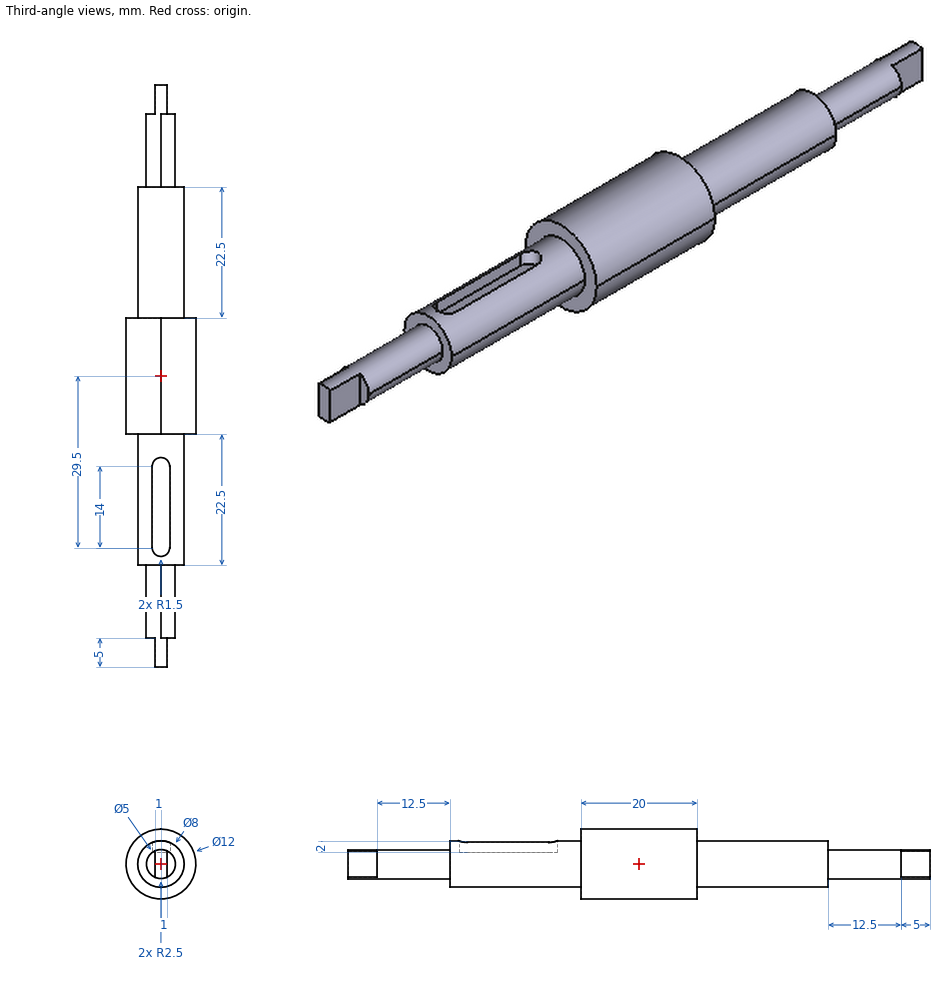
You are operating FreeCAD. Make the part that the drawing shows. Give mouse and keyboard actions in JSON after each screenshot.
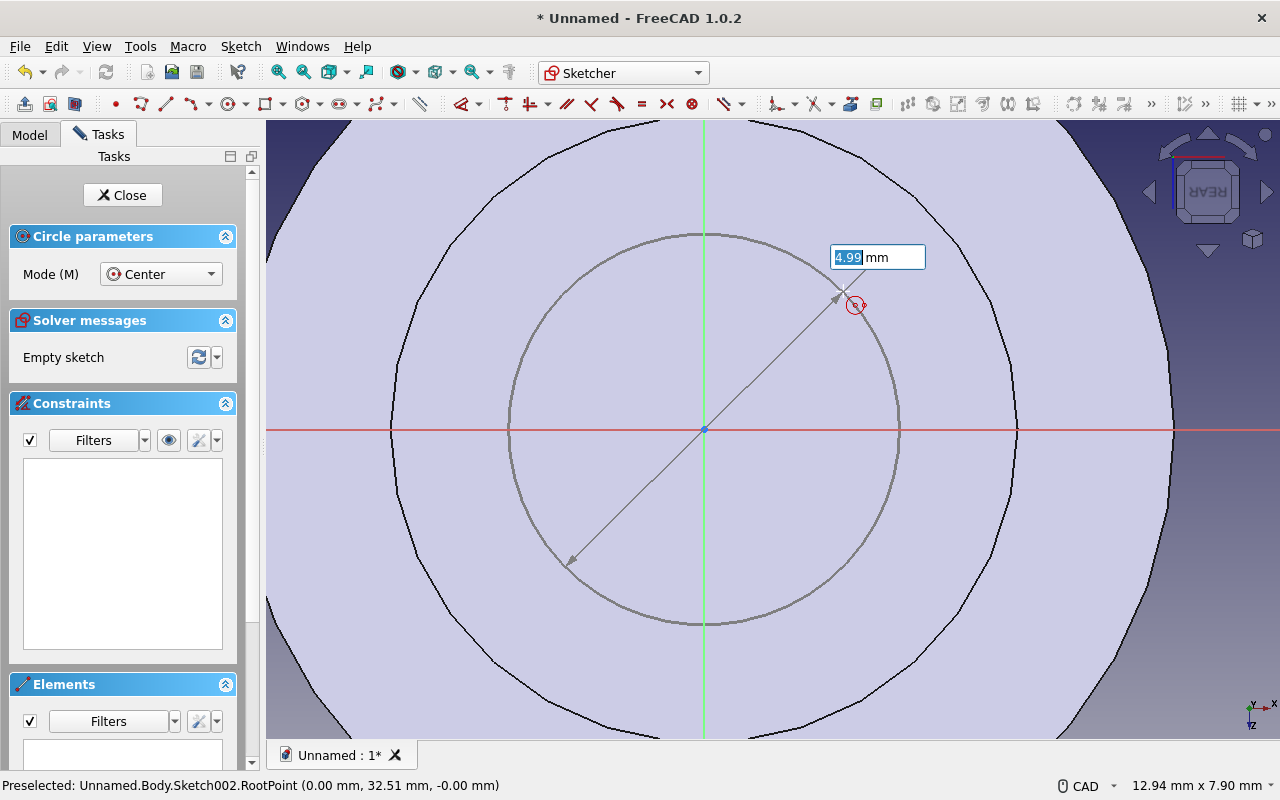
{"action": "type", "text": "5"}
{"action": "key", "text": "Return"}
{"action": "key", "text": "Escape"}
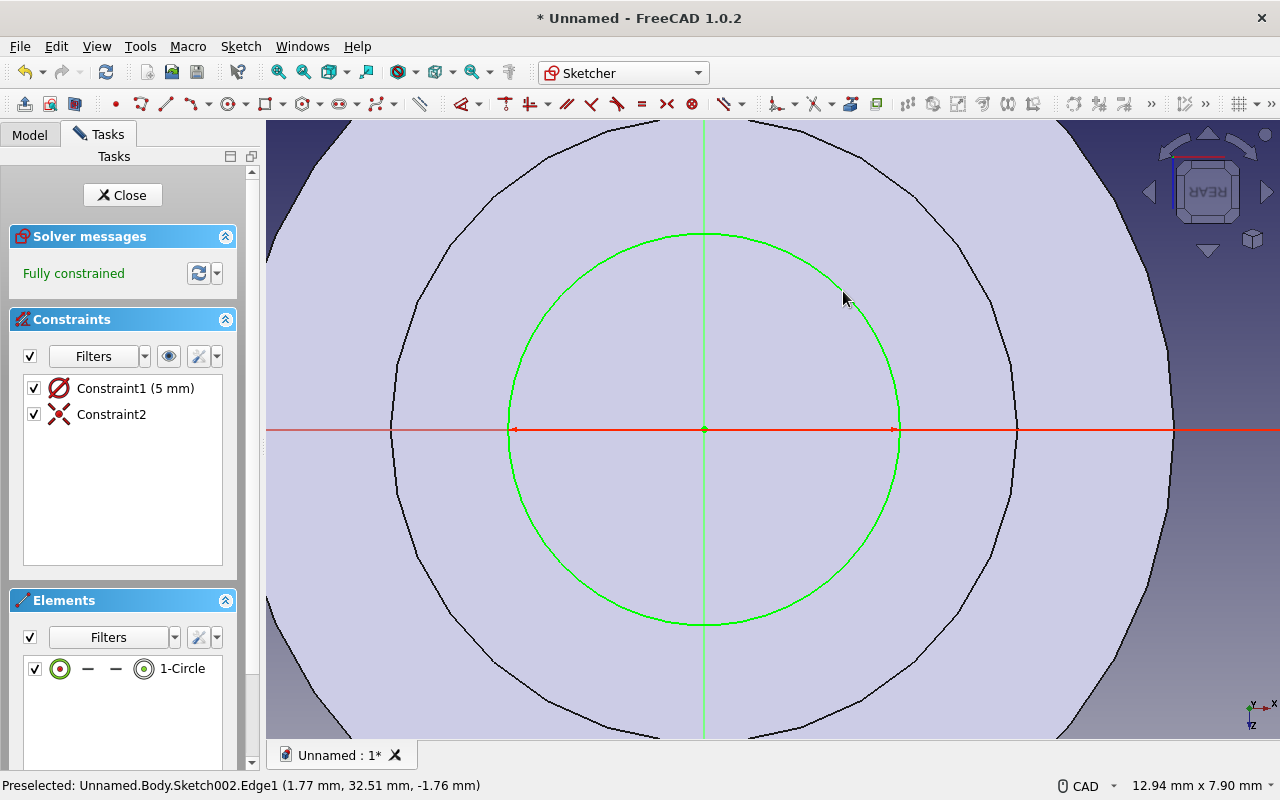
{"action": "left_click", "coordinate": [123, 195]}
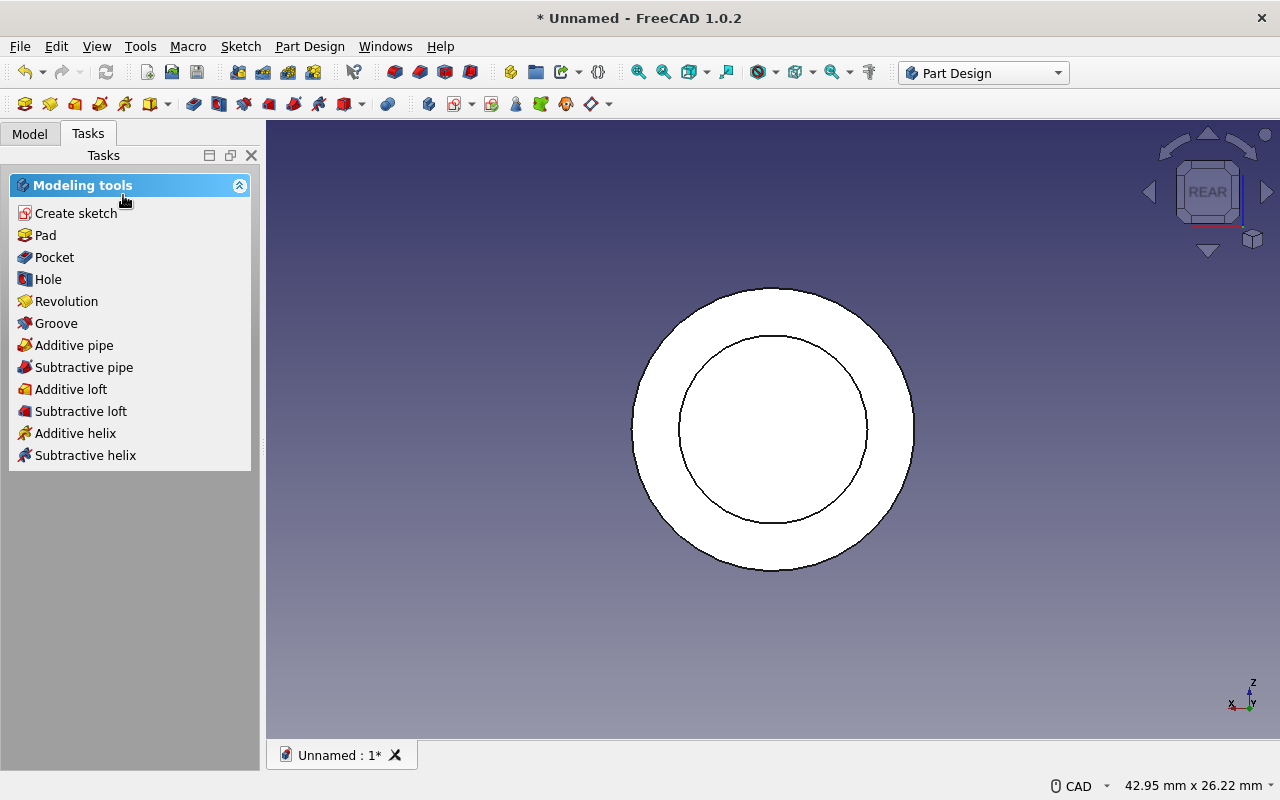
{"action": "left_click", "coordinate": [25, 104]}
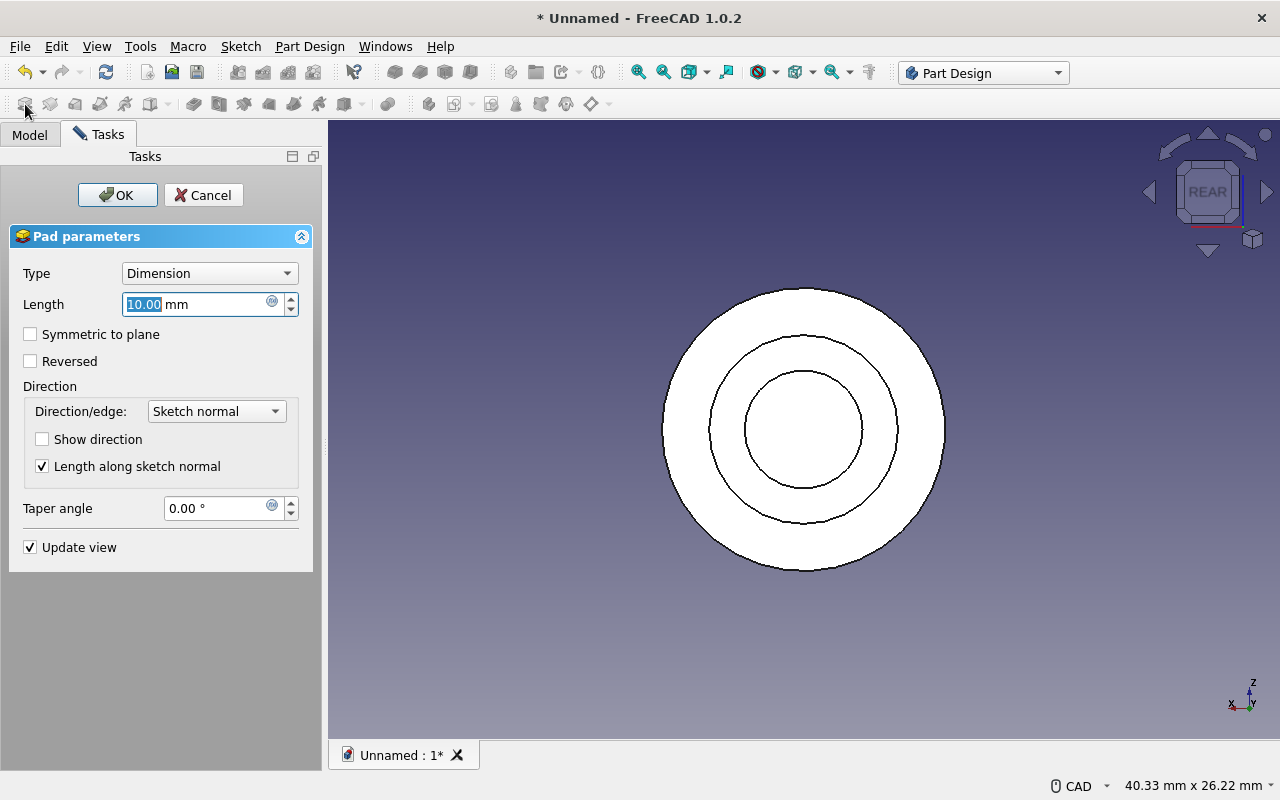
{"action": "type", "text": "12.5"}
{"action": "key", "text": "Tab"}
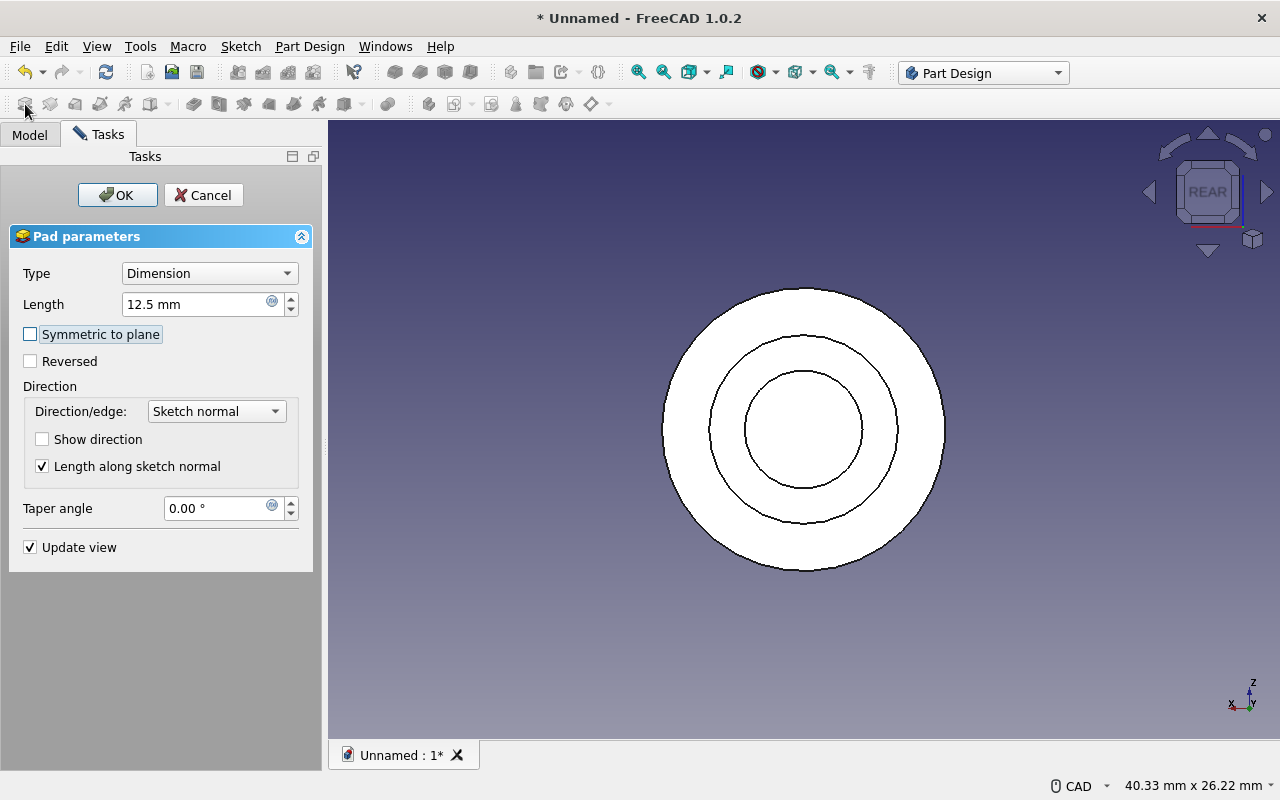
{"action": "left_click", "coordinate": [118, 195]}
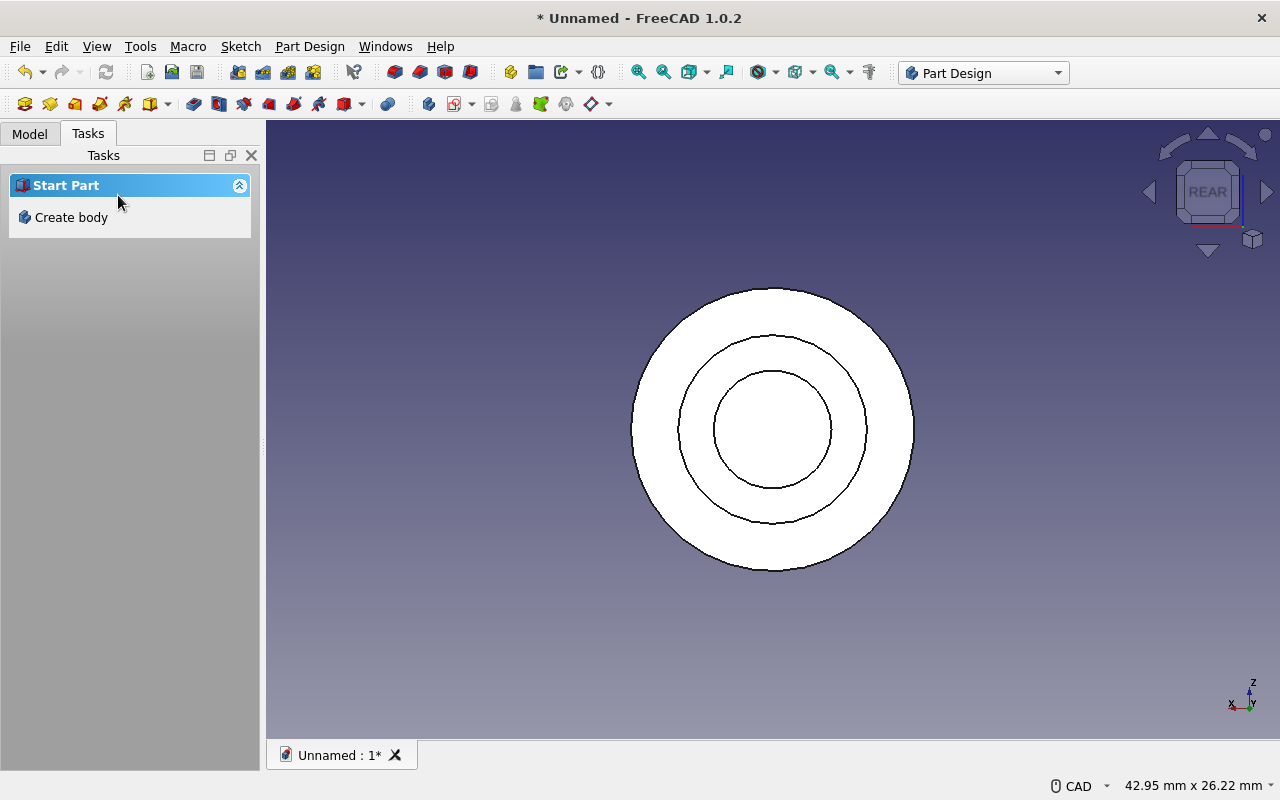
{"action": "left_click", "coordinate": [30, 134]}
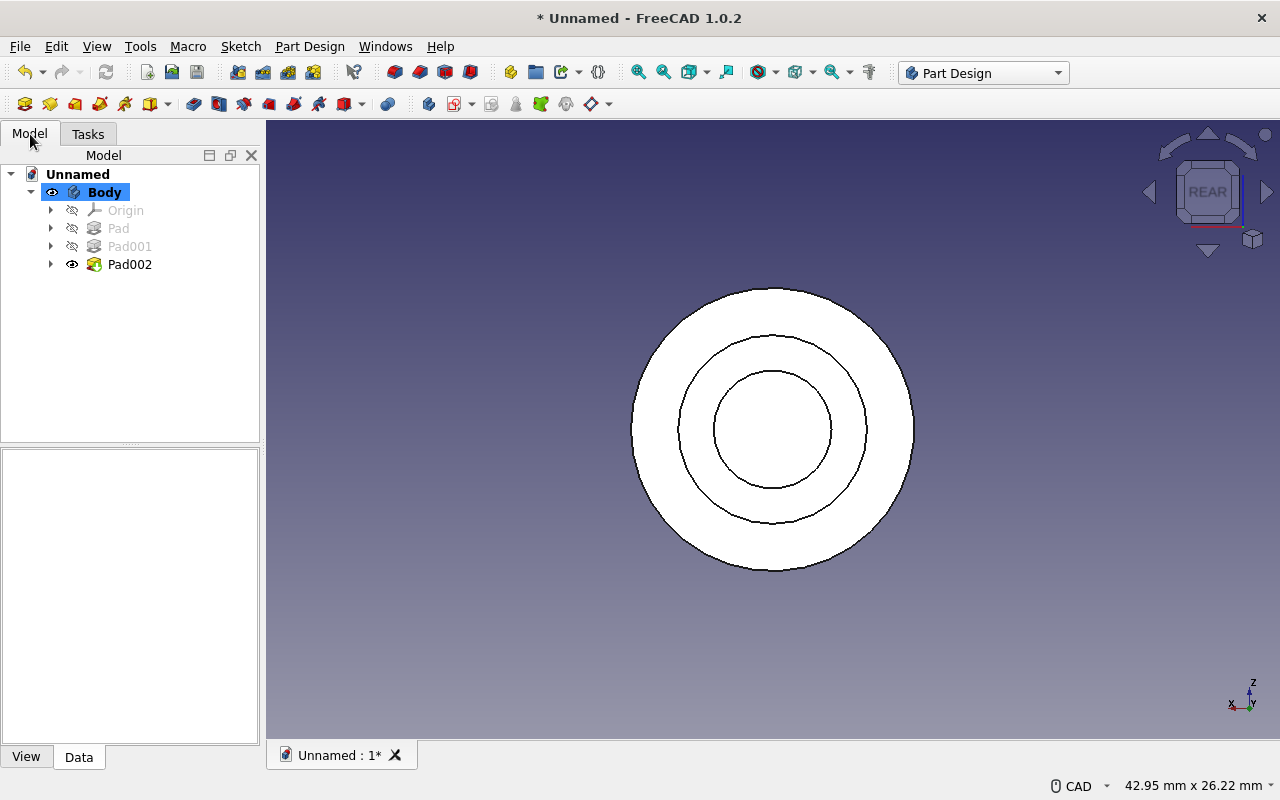
{"action": "left_click", "coordinate": [51, 210]}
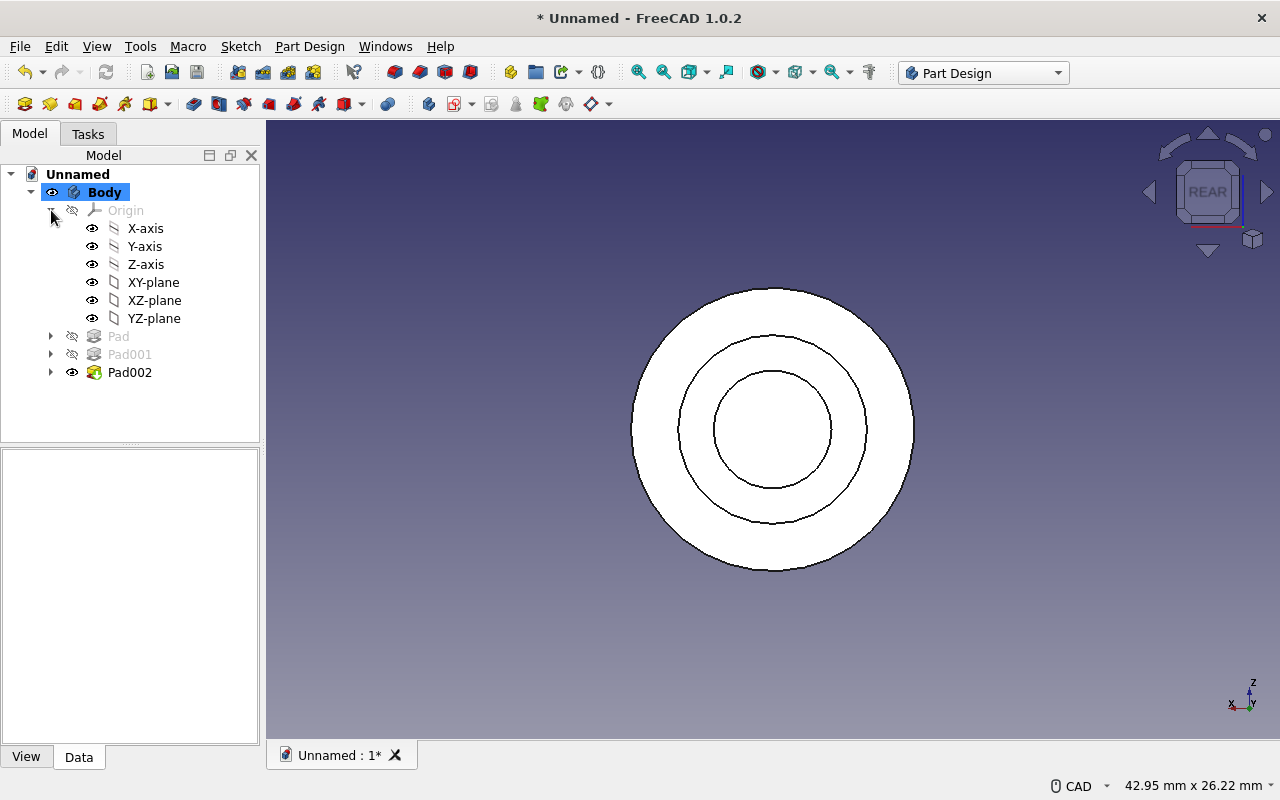
{"action": "left_click", "coordinate": [137, 300]}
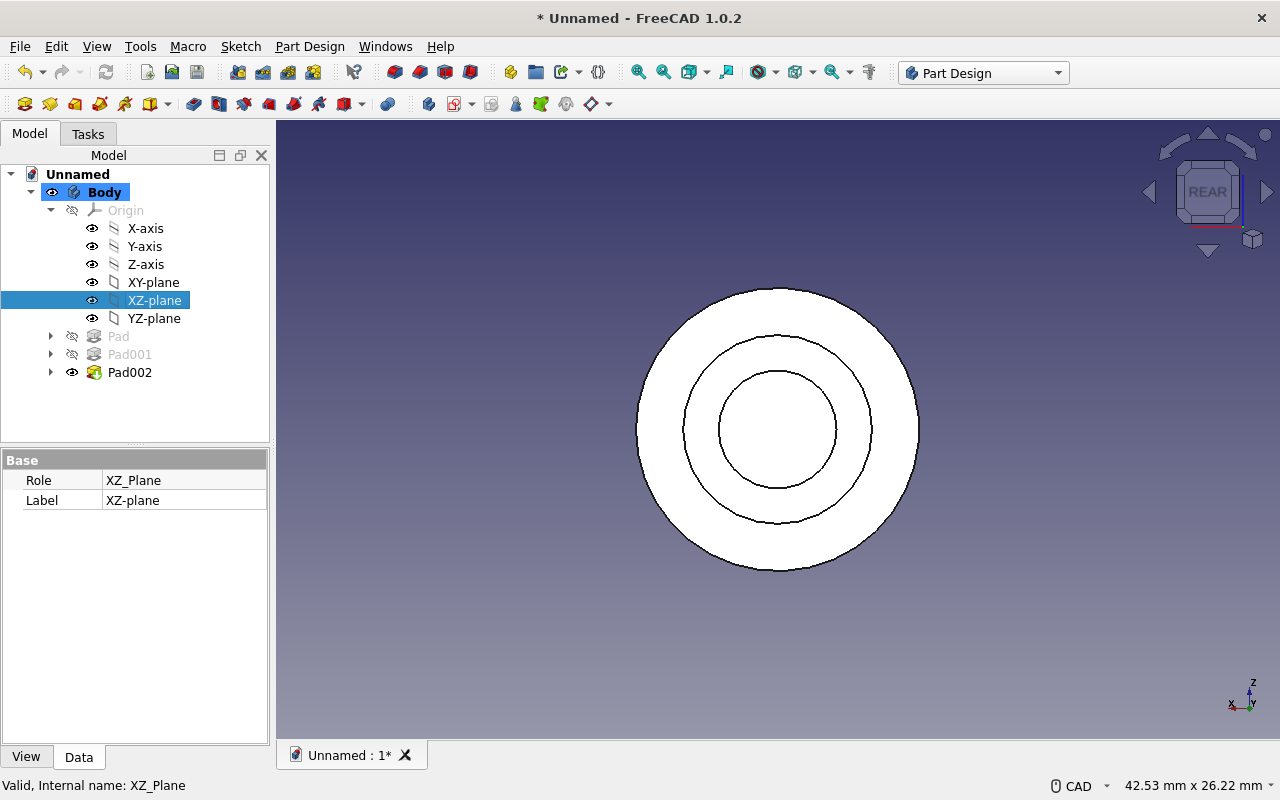
{"action": "left_click", "coordinate": [590, 104]}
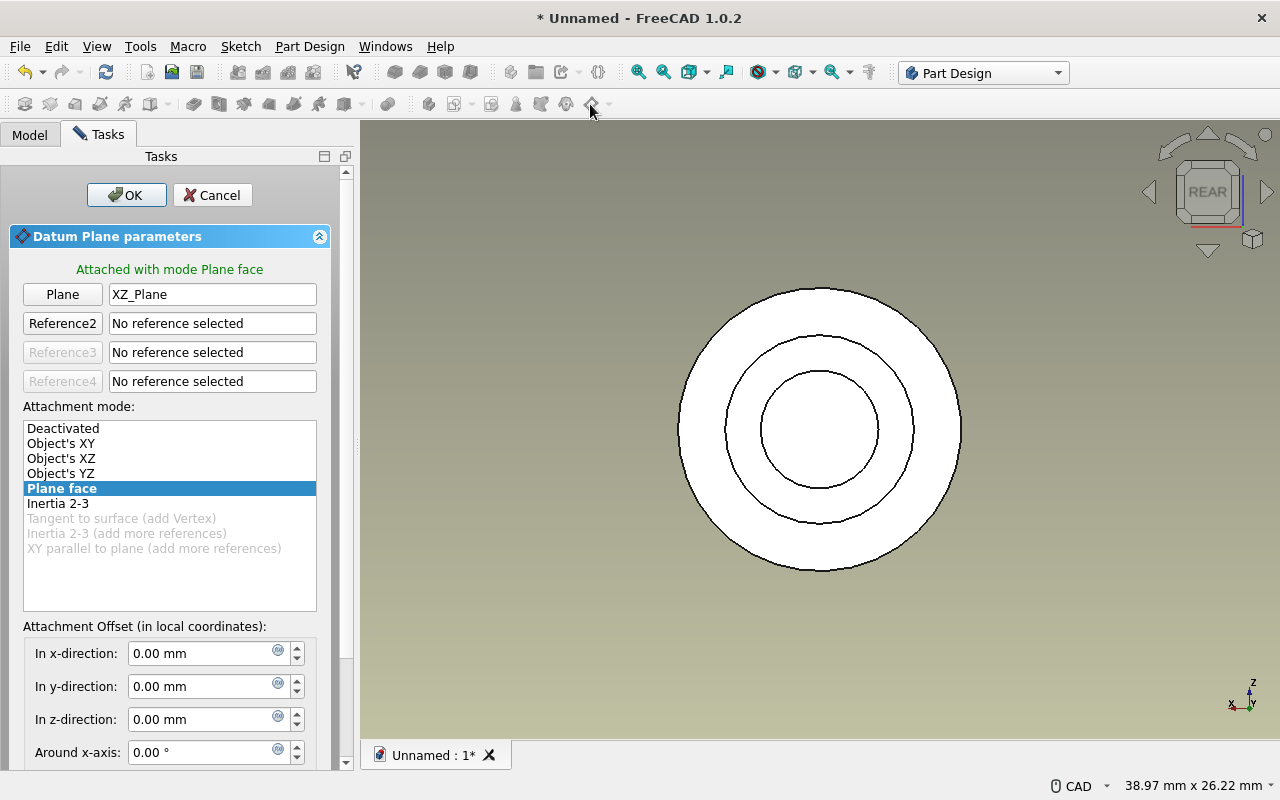
{"action": "triple_click", "coordinate": [210, 720]}